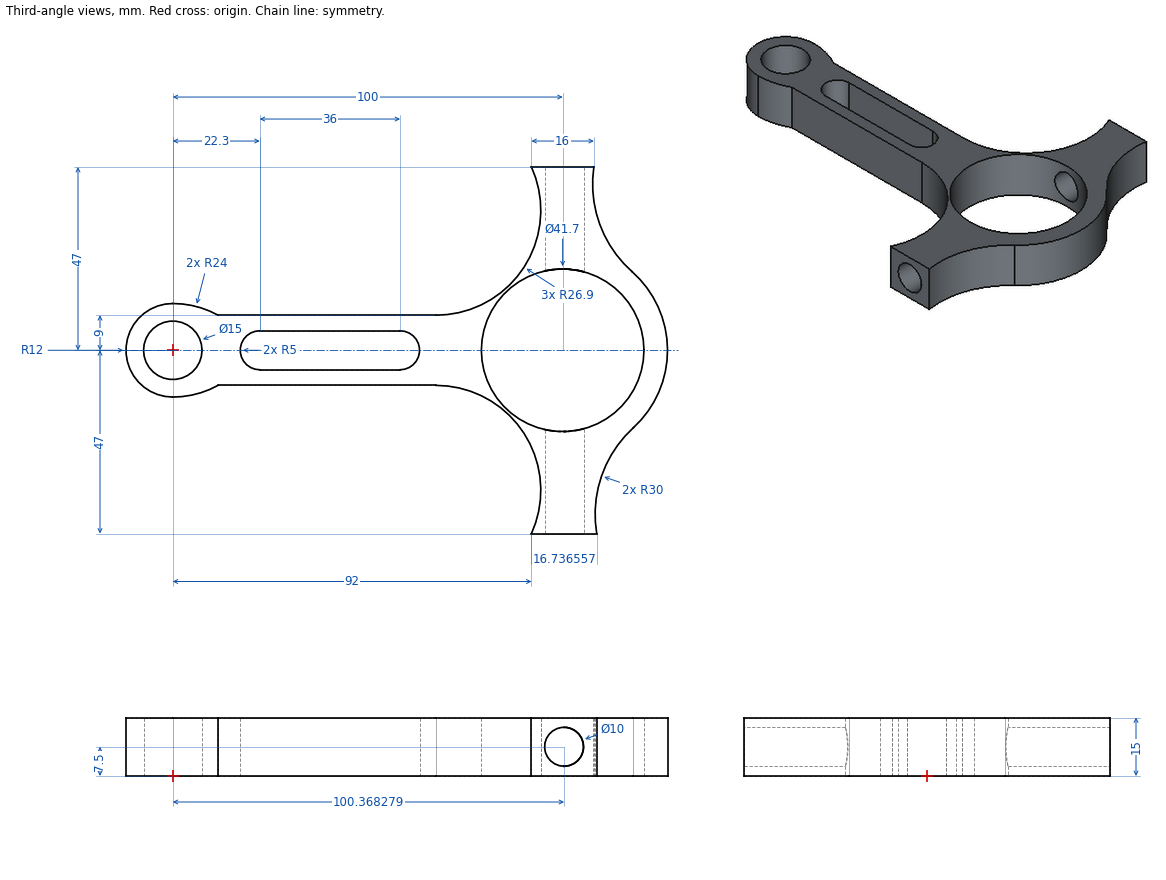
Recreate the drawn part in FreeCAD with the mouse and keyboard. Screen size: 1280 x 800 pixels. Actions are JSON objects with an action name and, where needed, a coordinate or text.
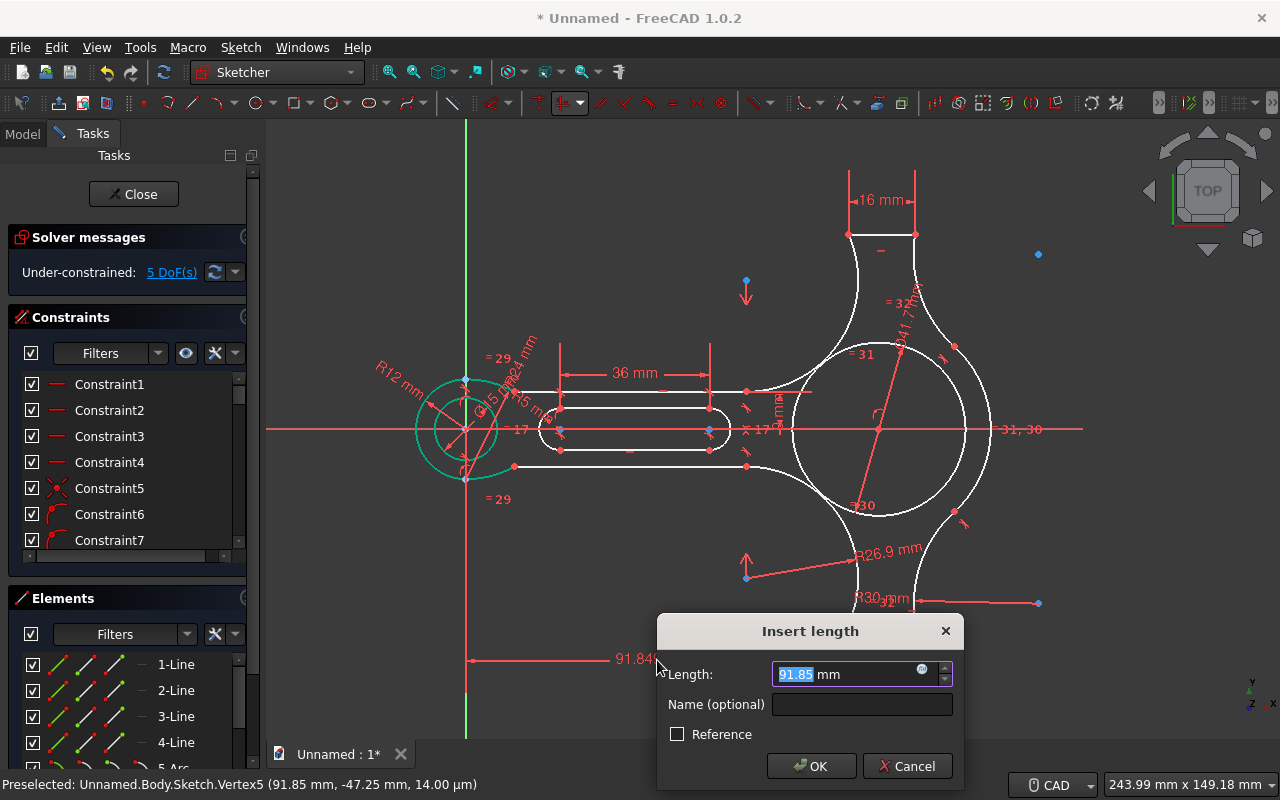
{"action": "type", "text": "92"}
{"action": "key", "text": "Return"}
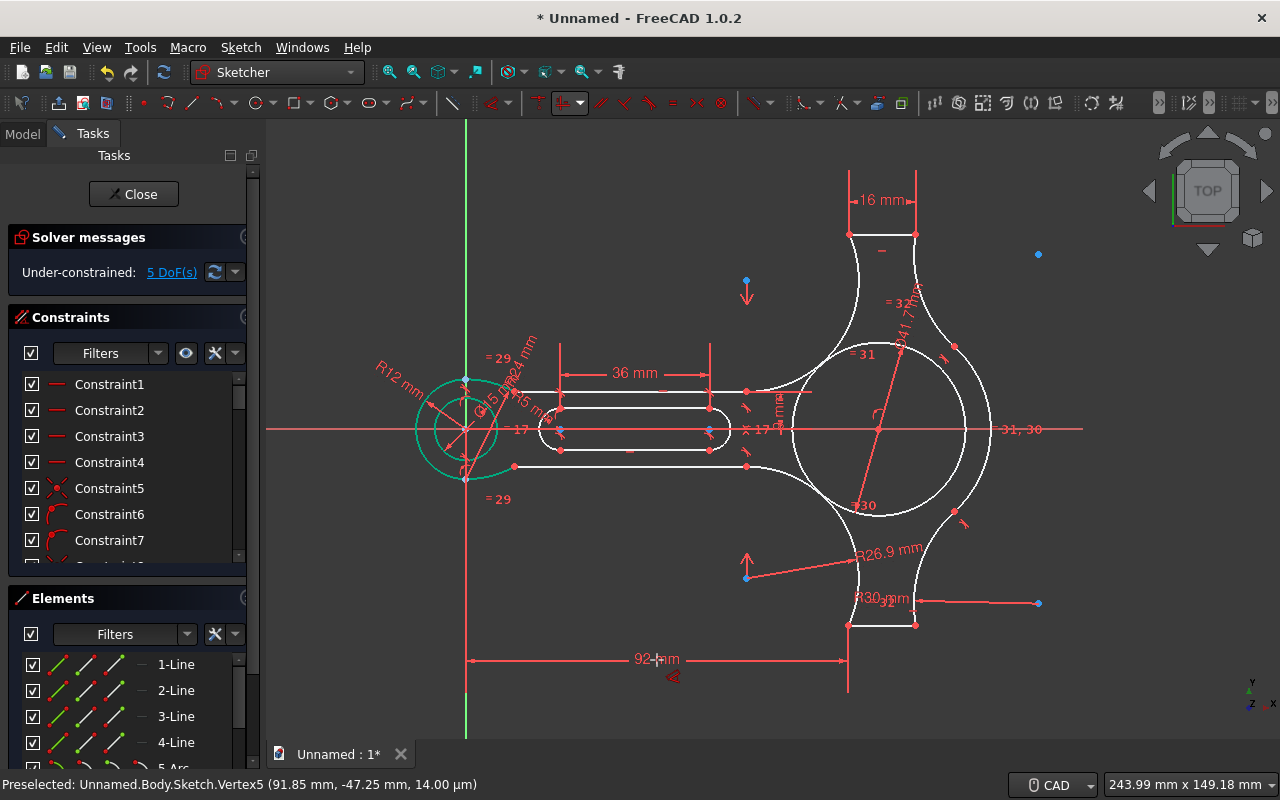
{"action": "left_click", "coordinate": [848, 626]}
{"action": "left_click", "coordinate": [432, 527]}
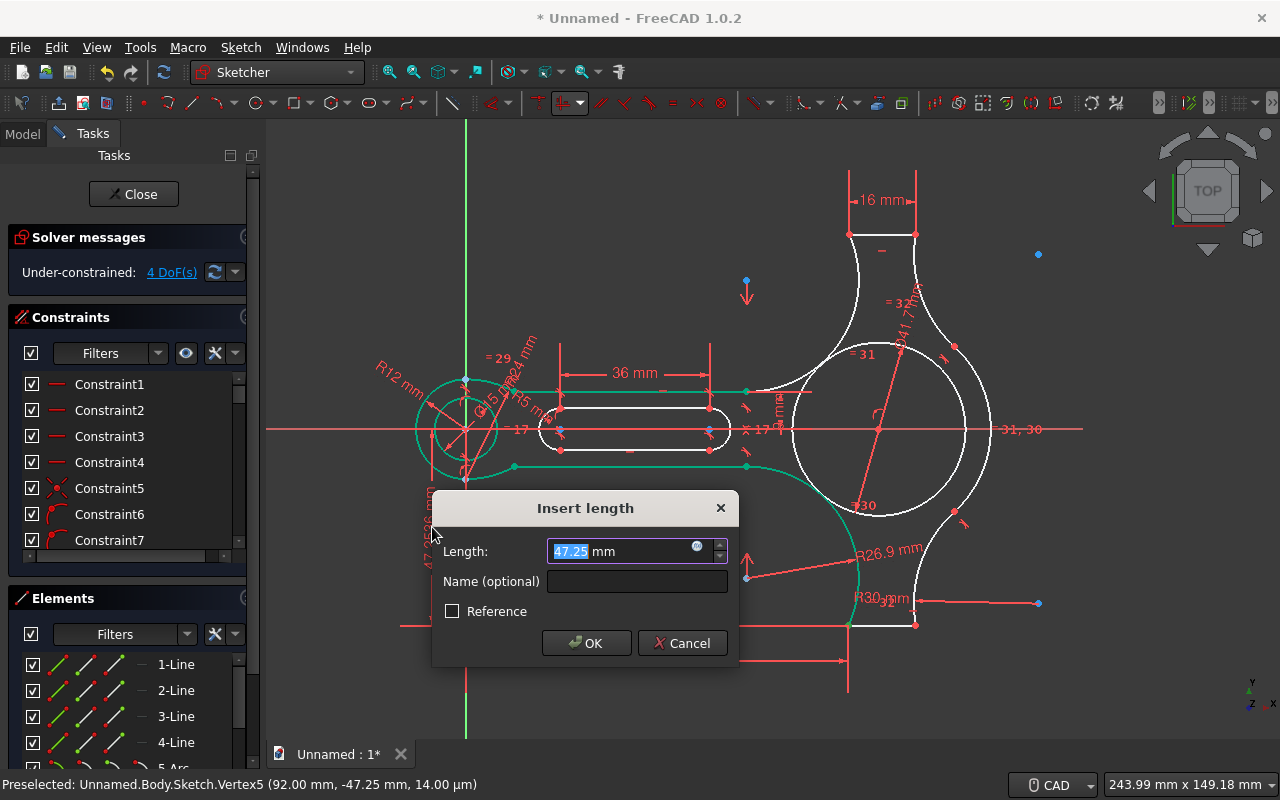
{"action": "type", "text": "47"}
{"action": "key", "text": "Return"}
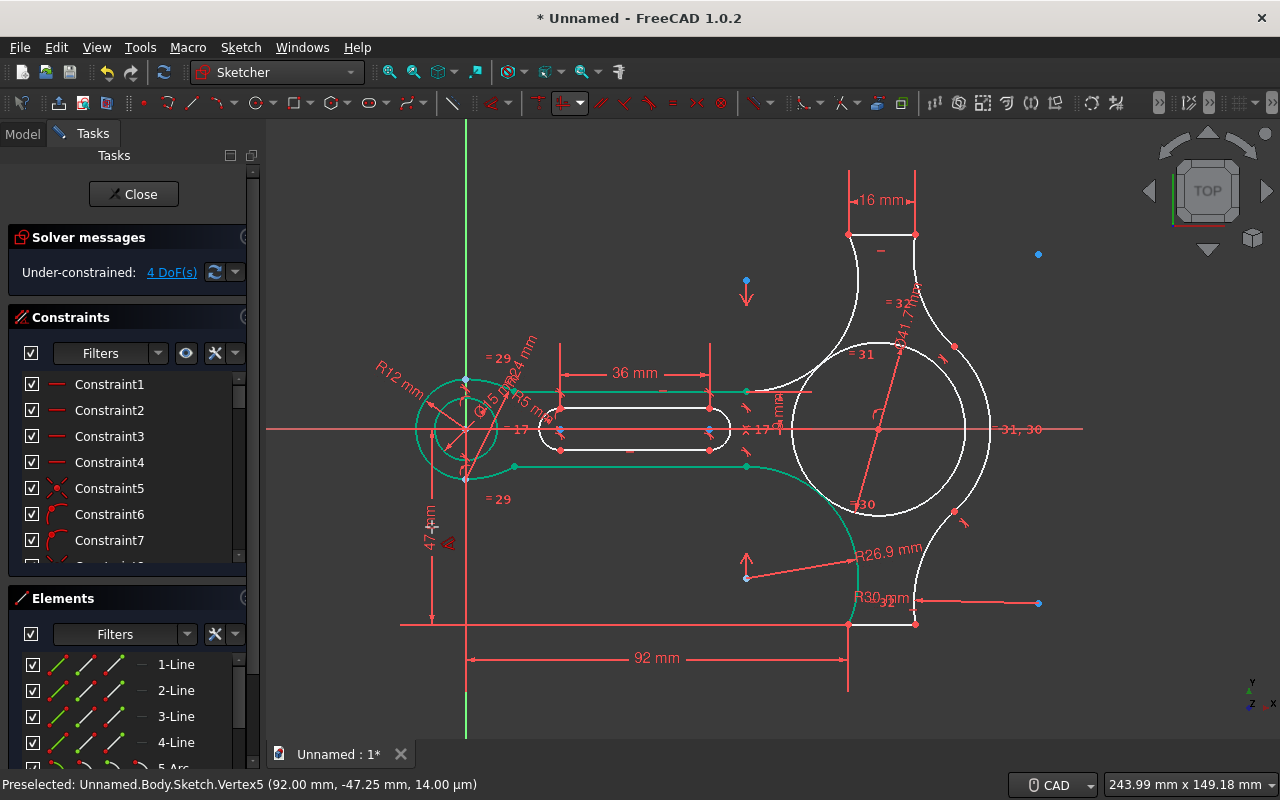
{"action": "left_click", "coordinate": [915, 235]}
{"action": "left_click", "coordinate": [432, 332]}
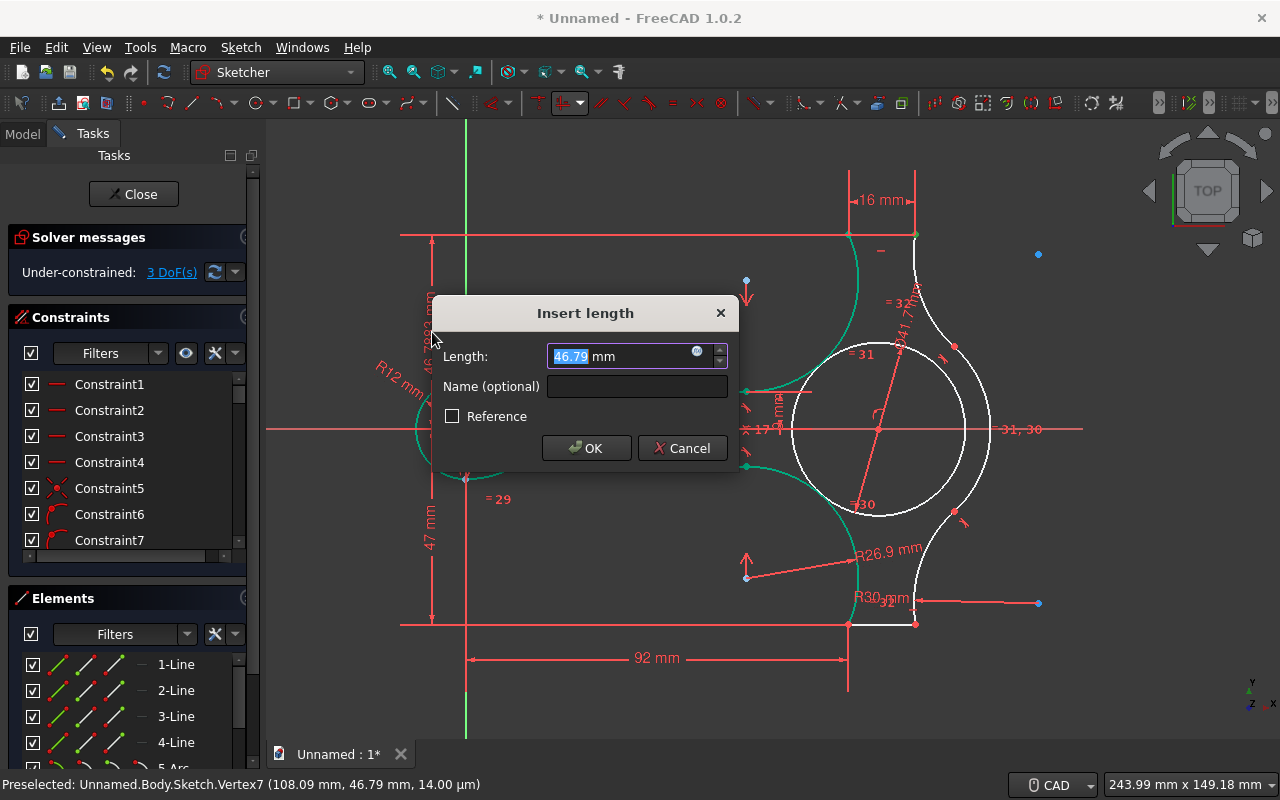
{"action": "type", "text": "47"}
{"action": "key", "text": "Return"}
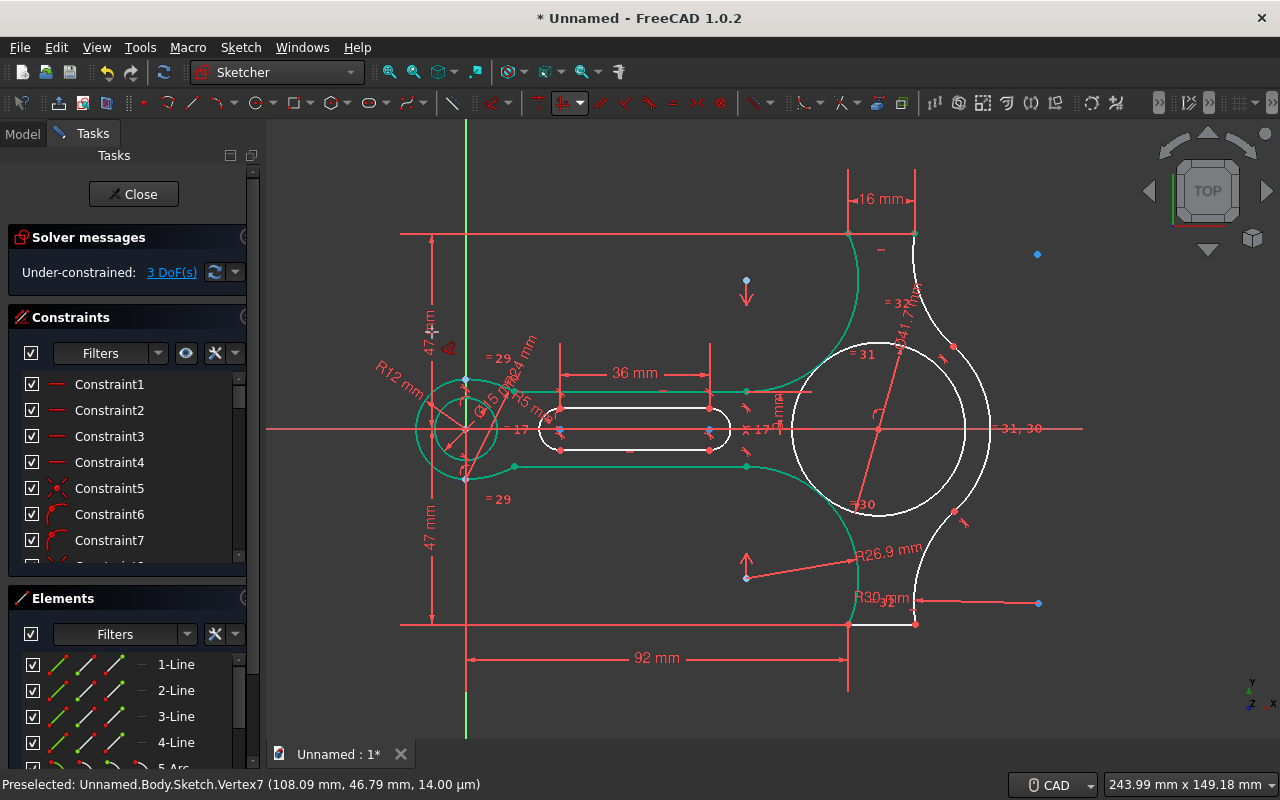
{"action": "left_click", "coordinate": [879, 429]}
{"action": "left_click", "coordinate": [817, 463]}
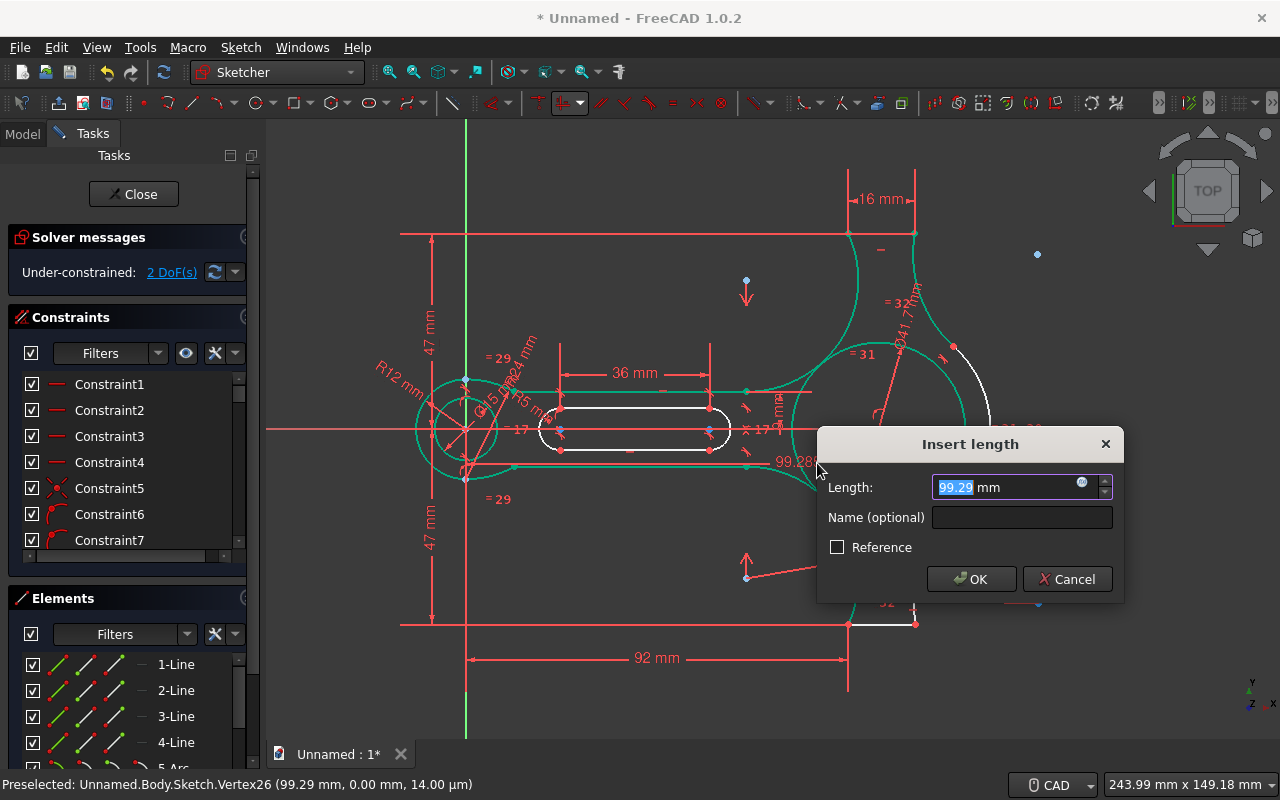
{"action": "type", "text": "100"}
{"action": "key", "text": "Return"}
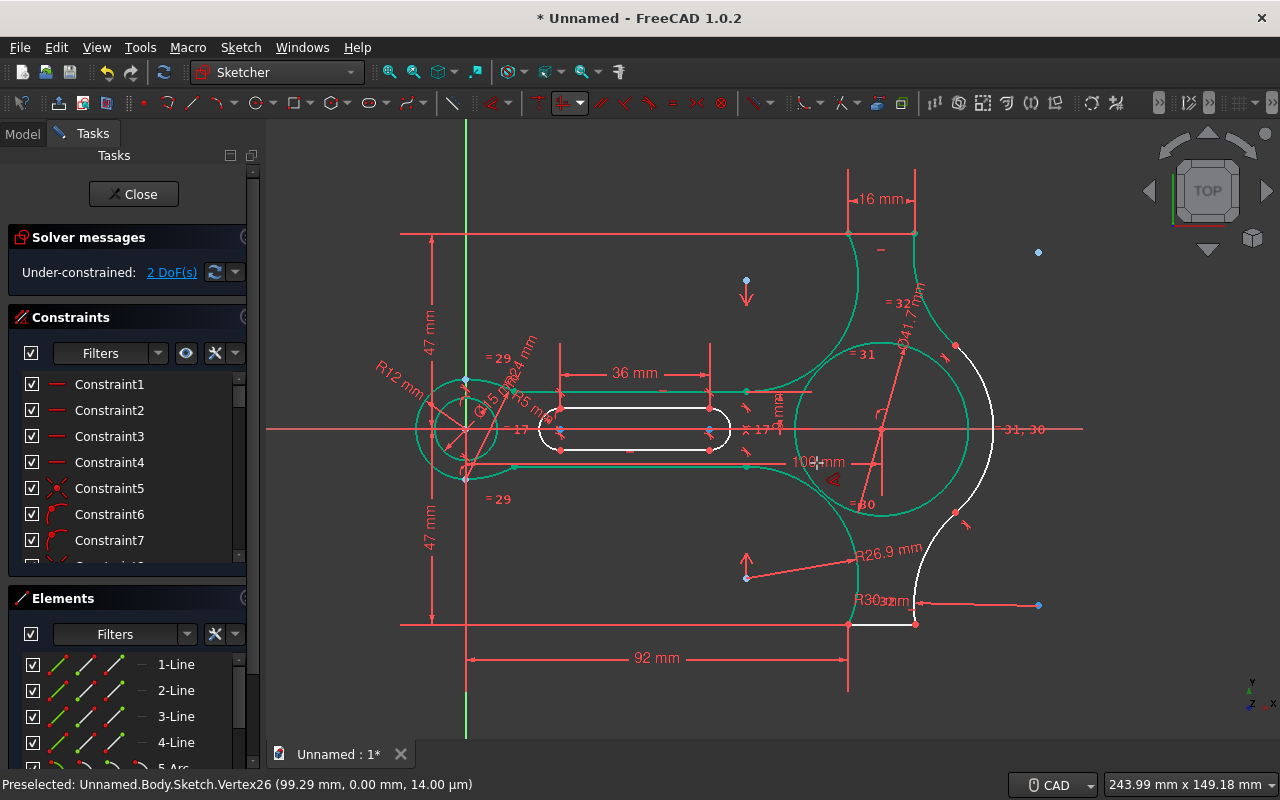
{"action": "left_click", "coordinate": [560, 408]}
{"action": "left_click", "coordinate": [513, 487]}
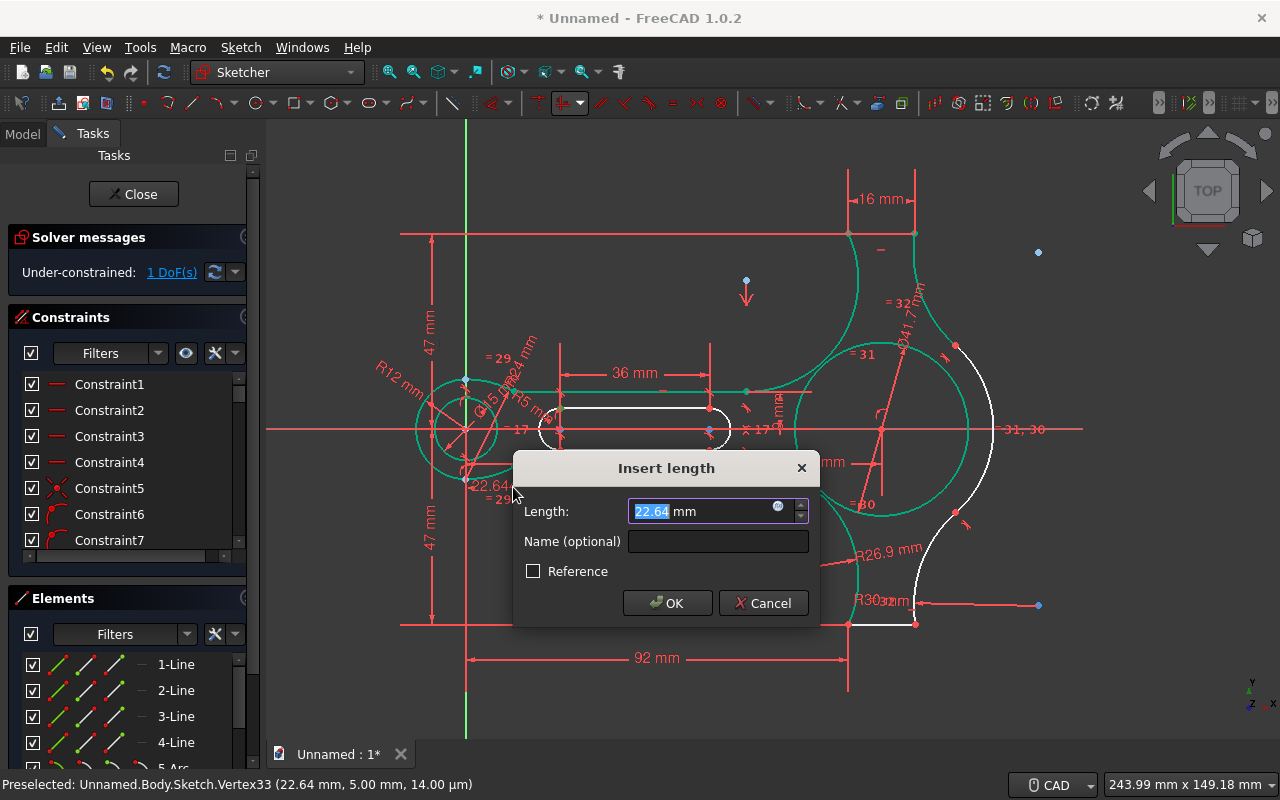
{"action": "type", "text": "22.3"}
{"action": "key", "text": "Return"}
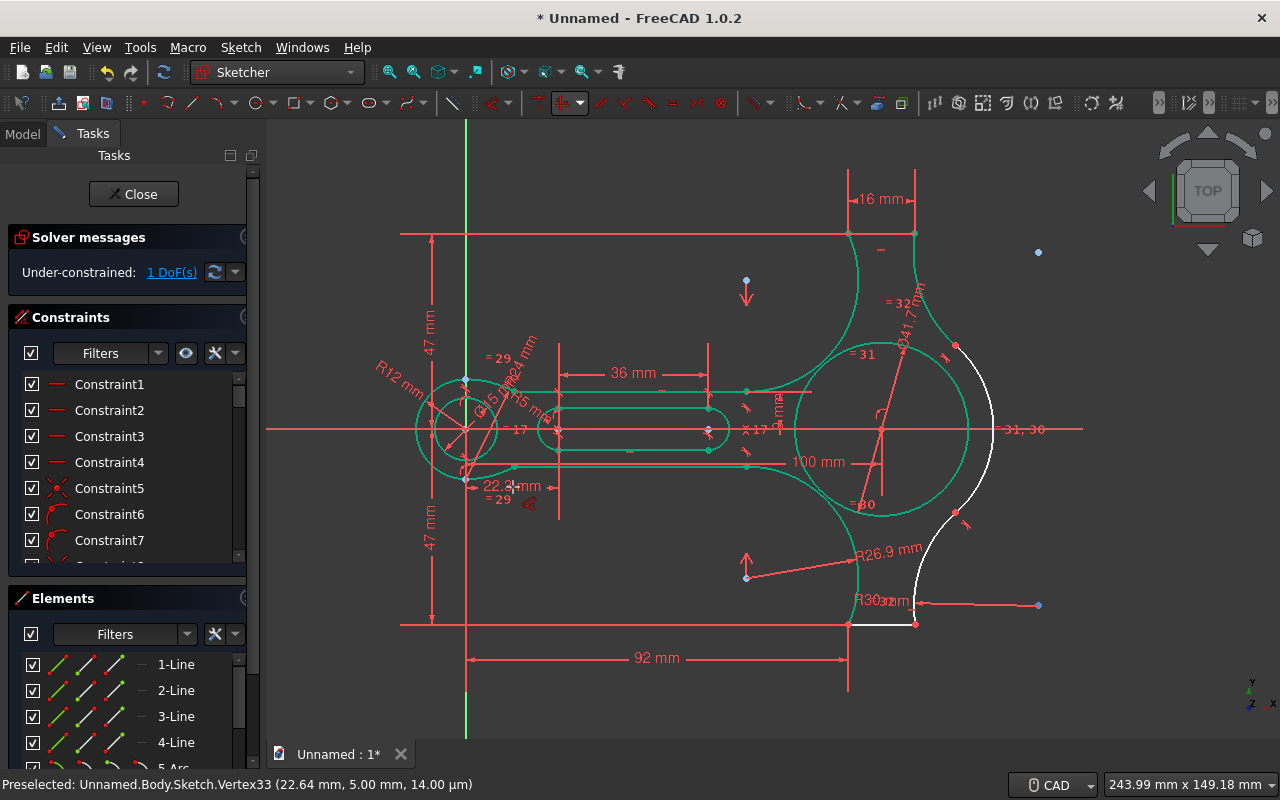
{"action": "left_click", "coordinate": [868, 625]}
{"action": "left_click", "coordinate": [882, 659]}